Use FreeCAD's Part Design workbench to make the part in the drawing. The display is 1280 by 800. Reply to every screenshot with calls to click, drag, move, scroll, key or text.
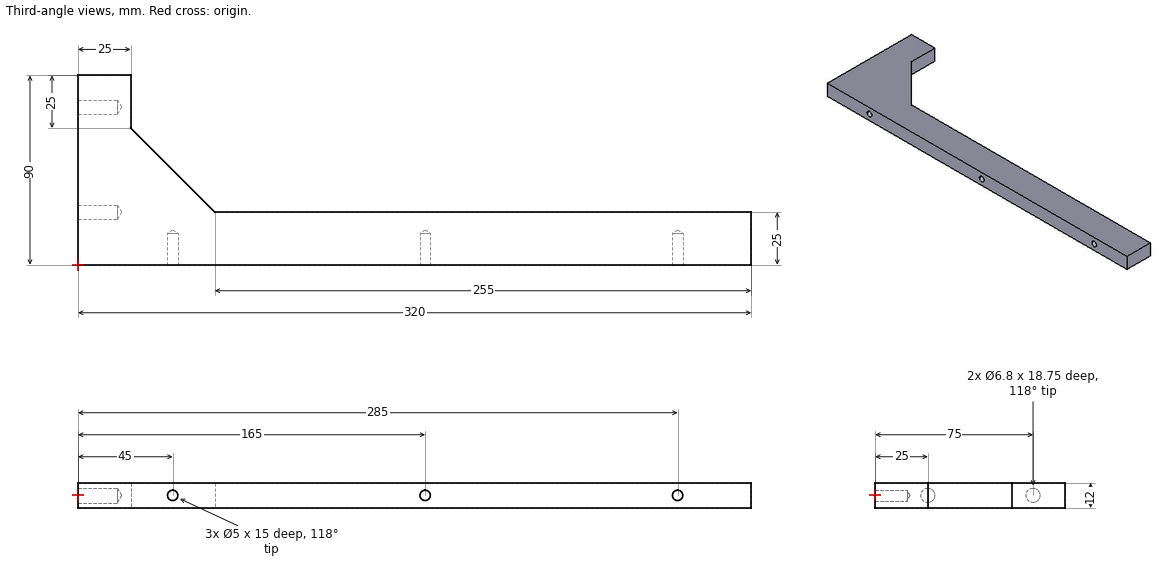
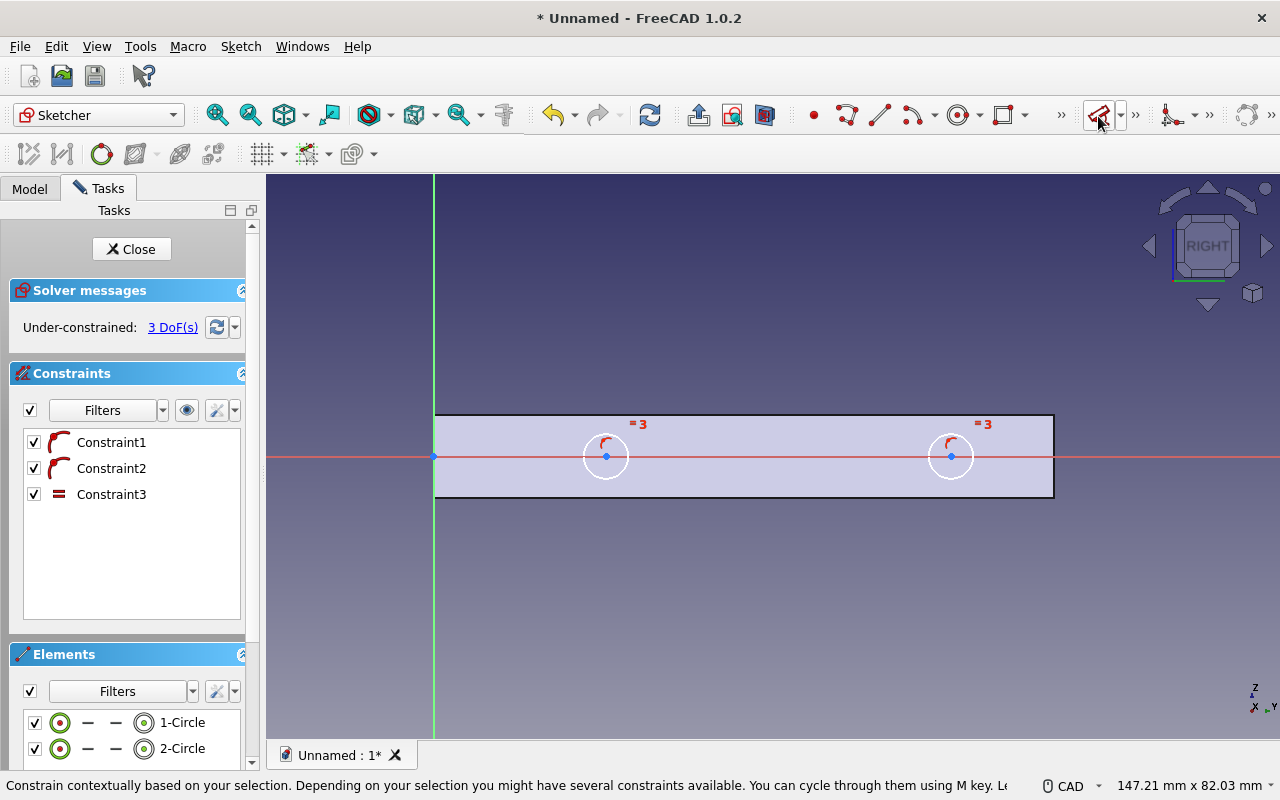
click(967, 441)
click(990, 419)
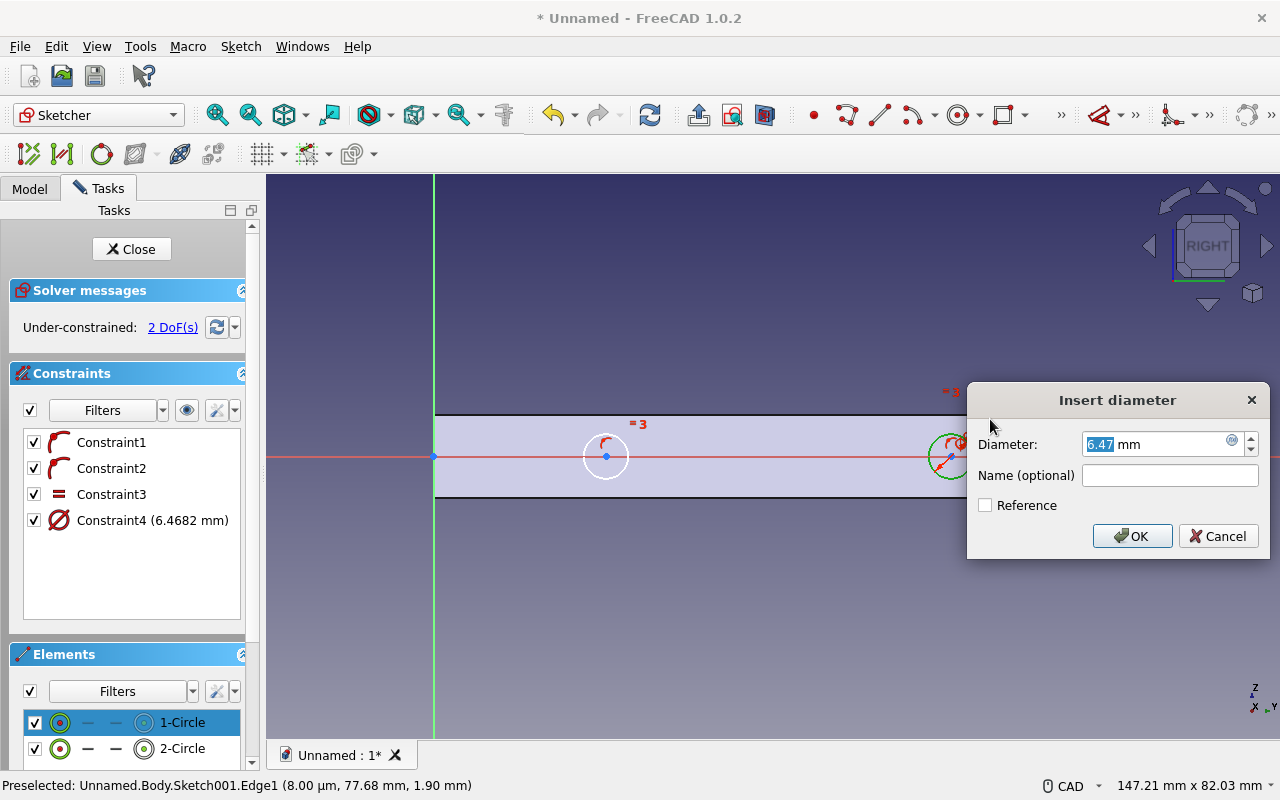
text(6.8)
key(Return)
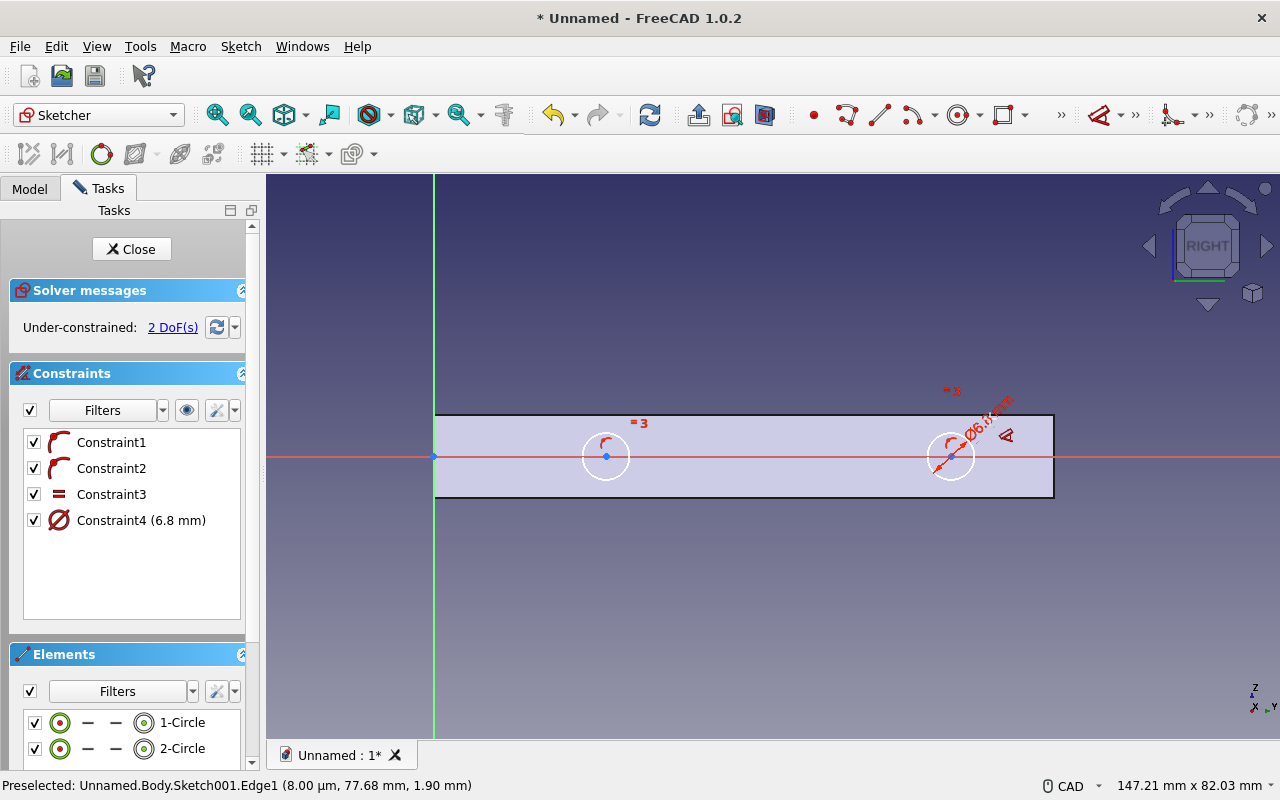
click(951, 456)
click(692, 490)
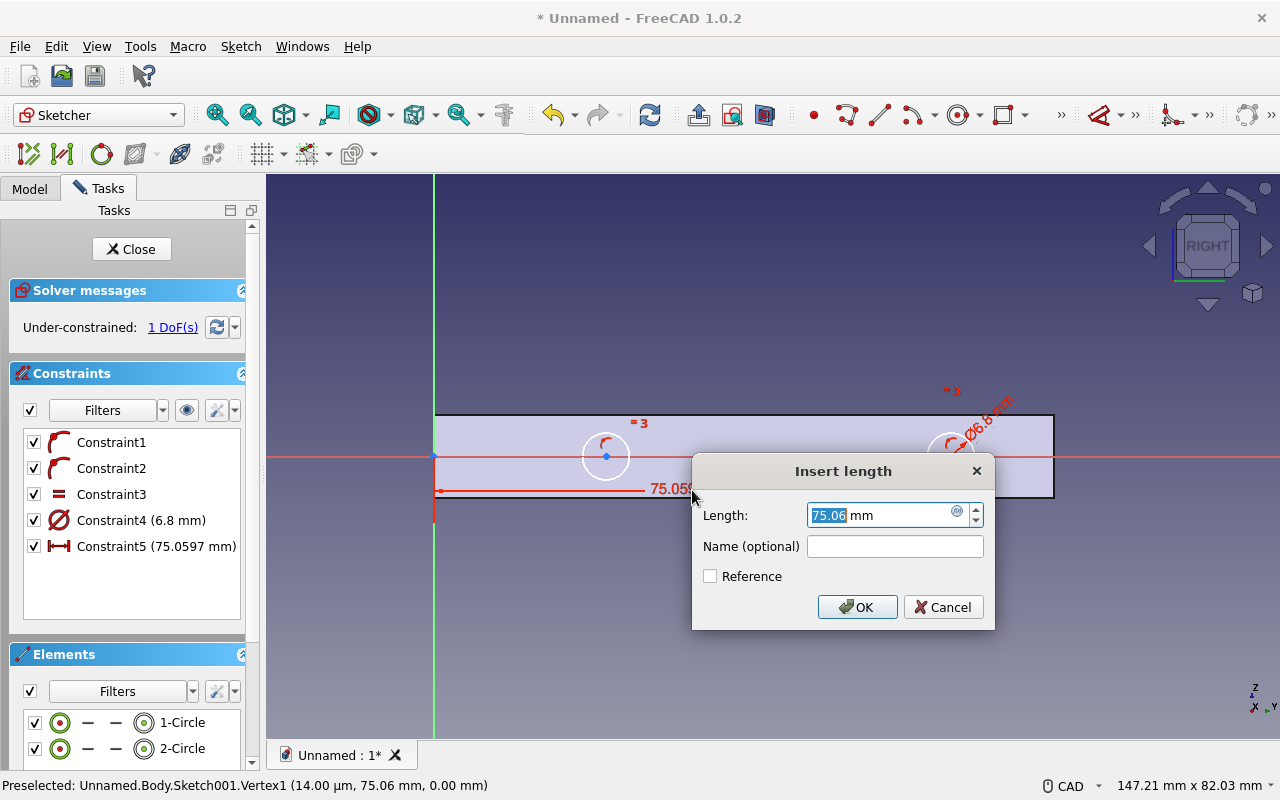
text(75)
key(Return)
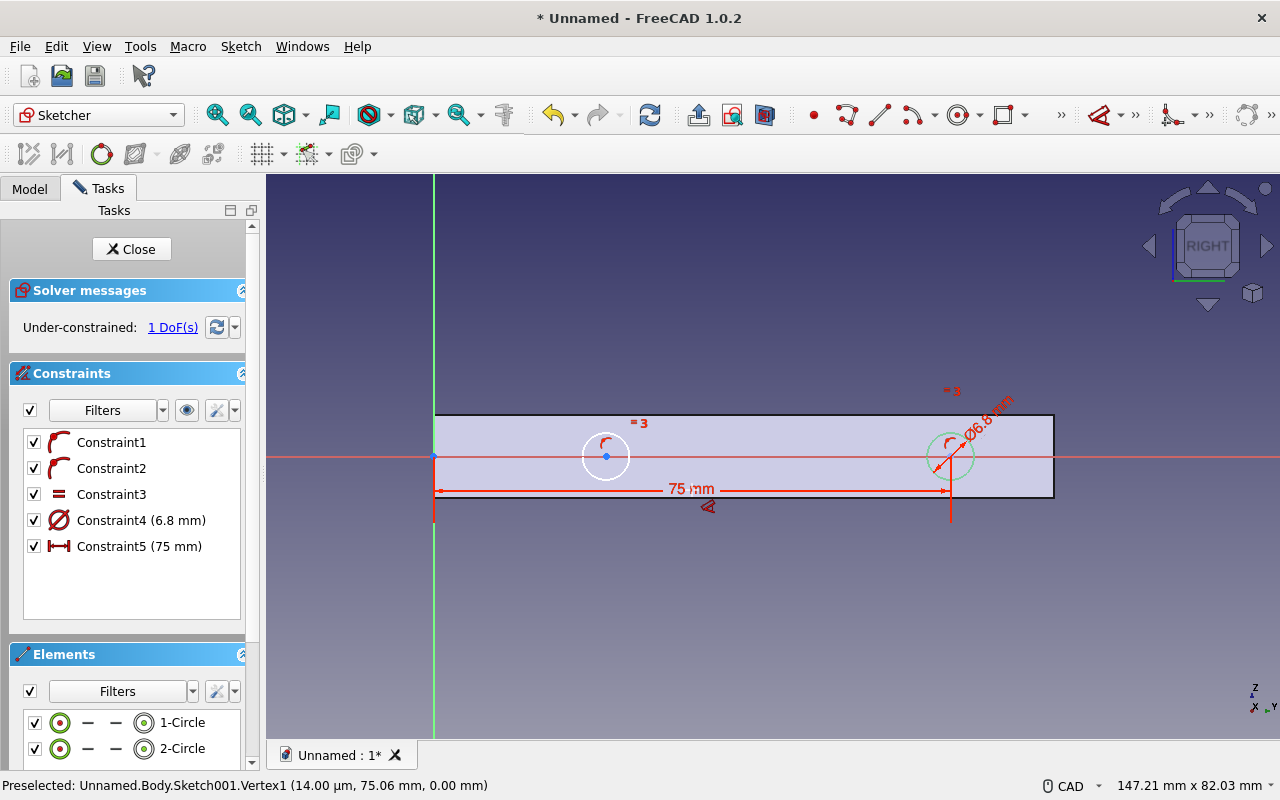
click(606, 456)
click(520, 490)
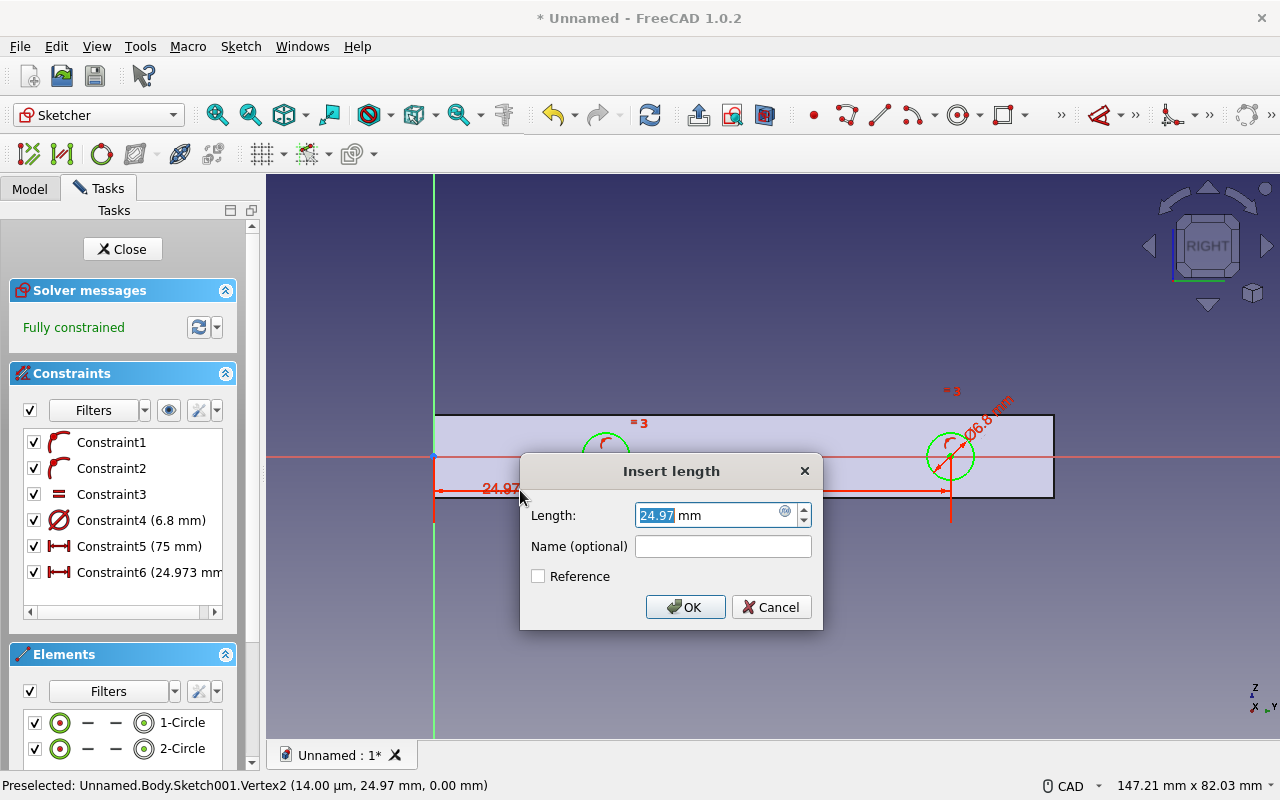
text(25)
key(Return)
key(Escape)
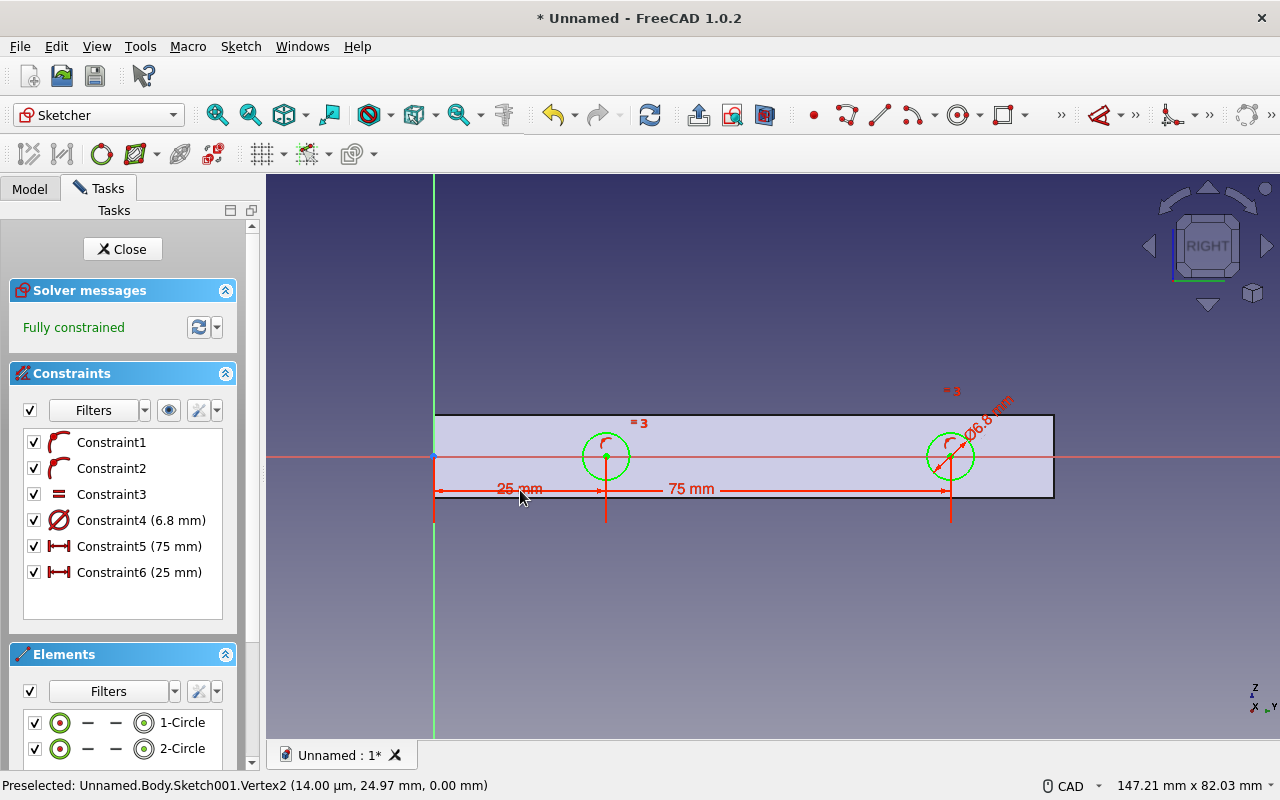
click(123, 249)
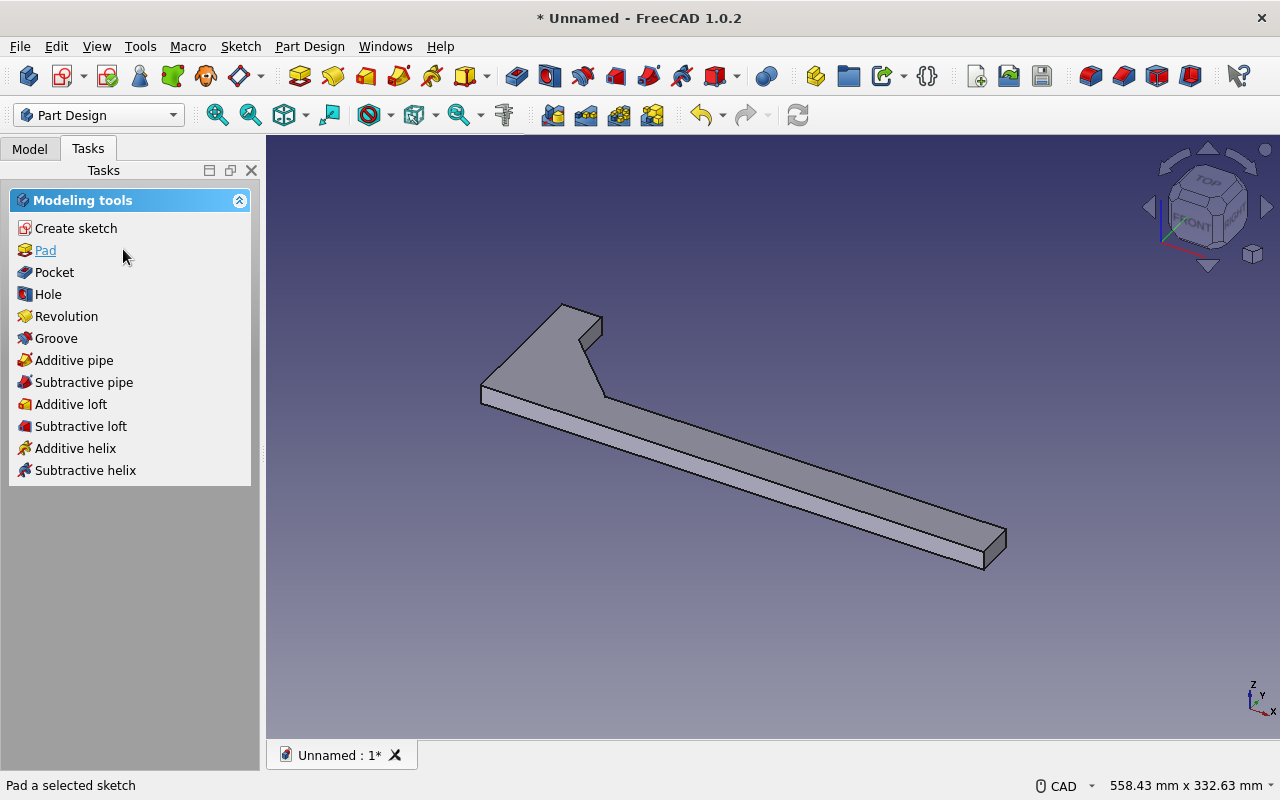
click(550, 76)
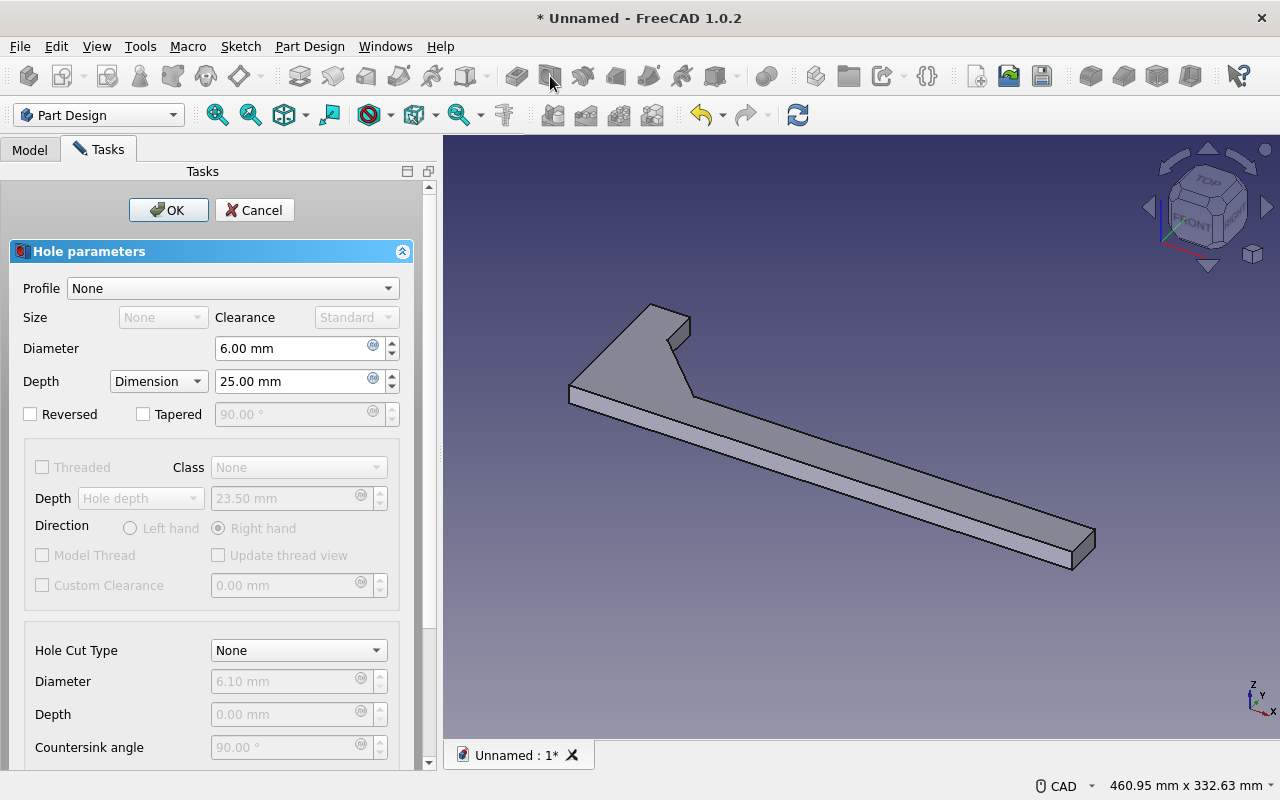
triple_click(300, 348)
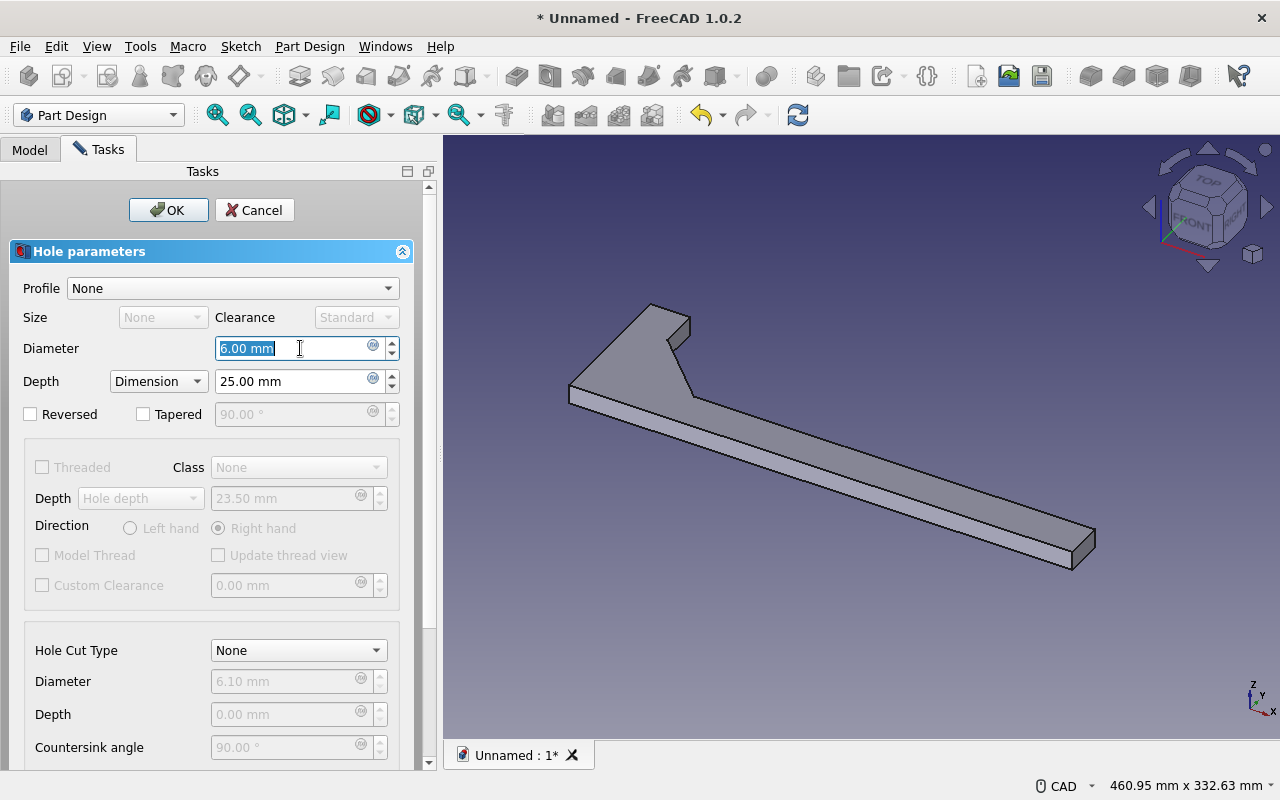
text(6.8)
key(Tab)